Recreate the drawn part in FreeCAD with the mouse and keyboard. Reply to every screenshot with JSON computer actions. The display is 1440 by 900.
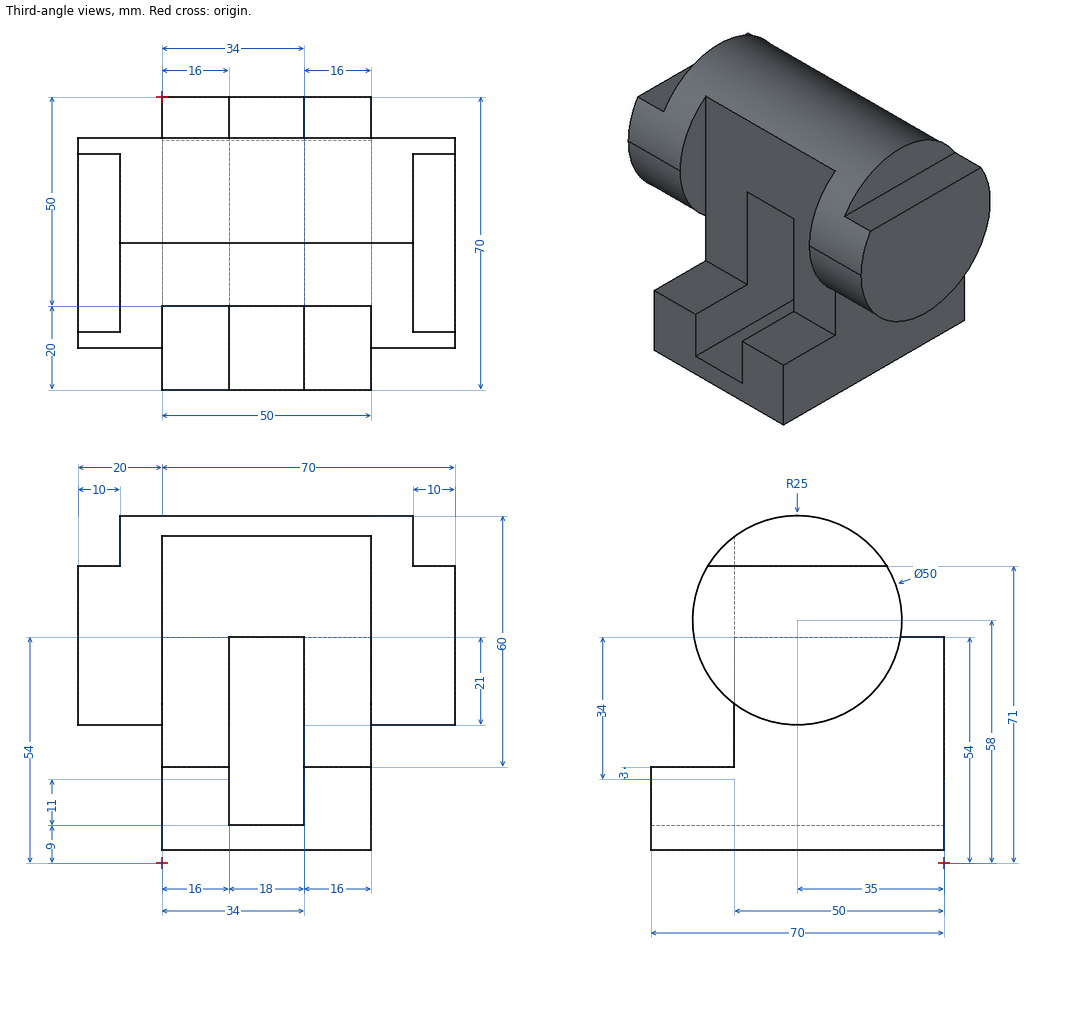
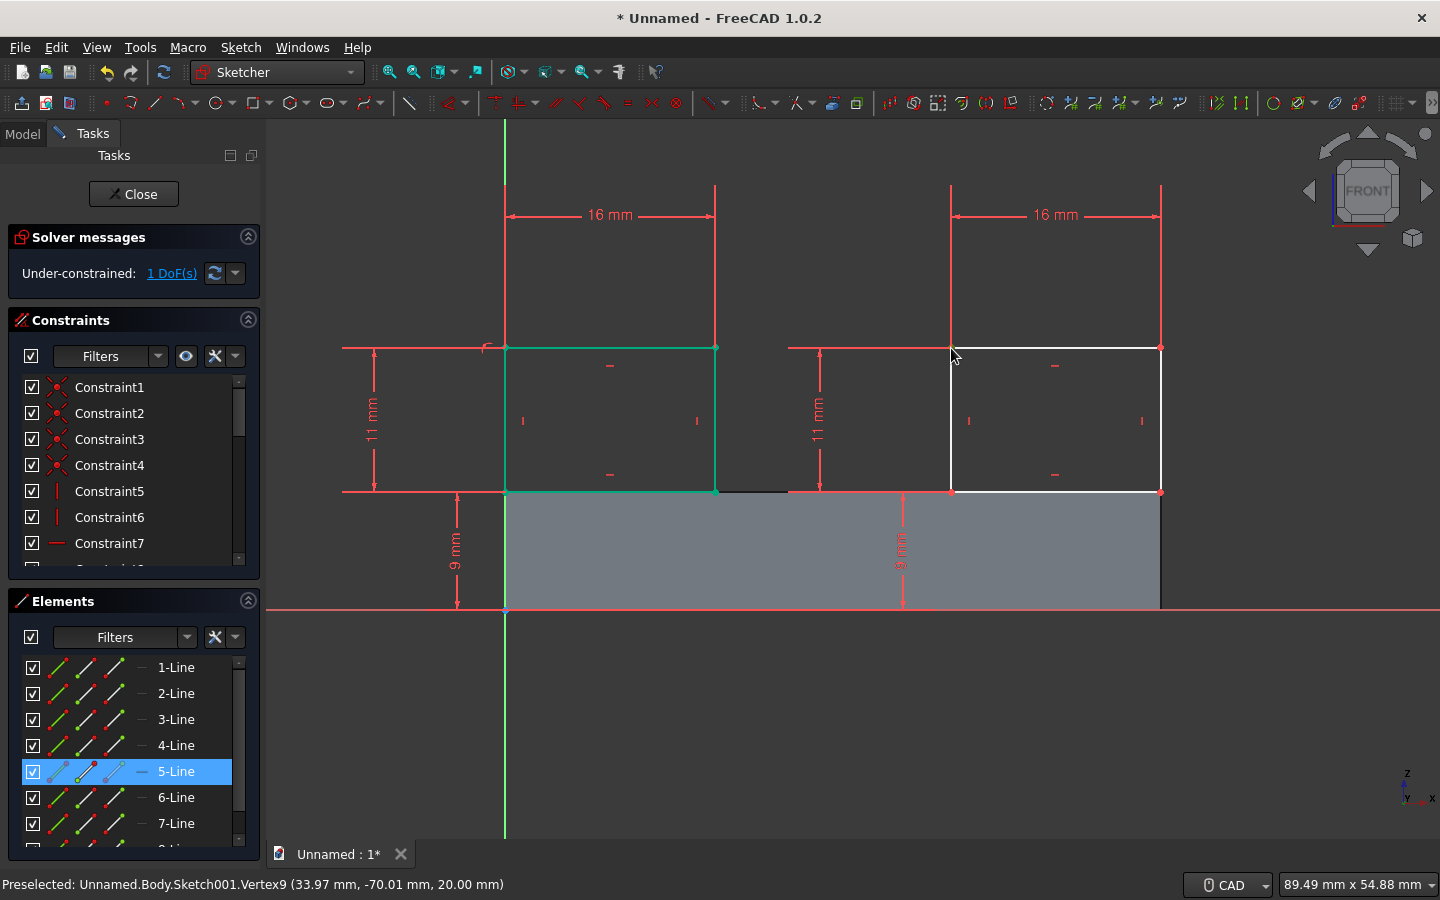
{"action": "key", "text": "l"}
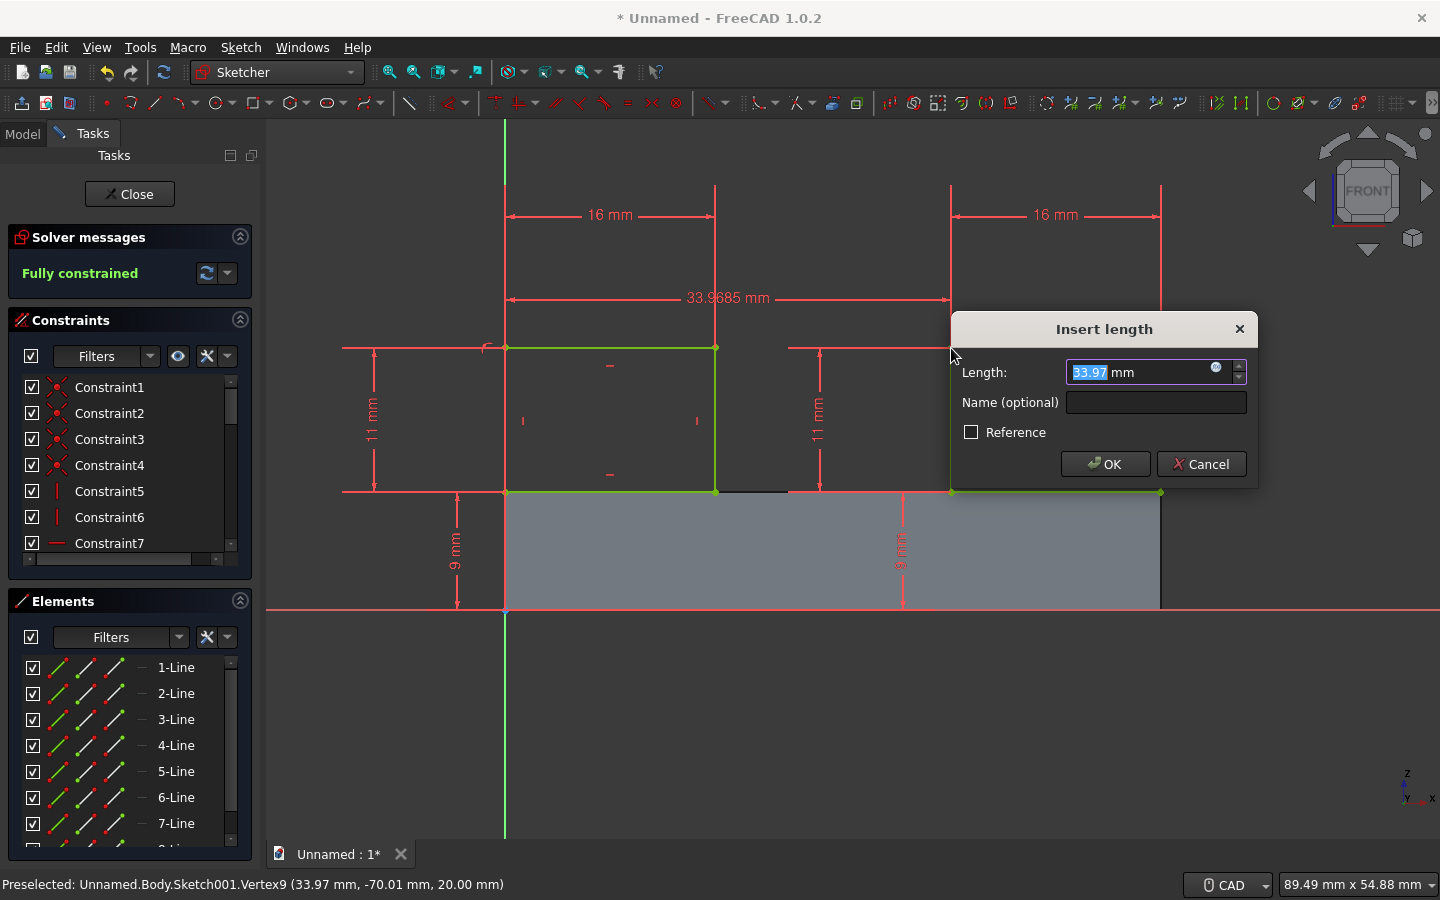
{"action": "type", "text": "34"}
{"action": "key", "text": "Return"}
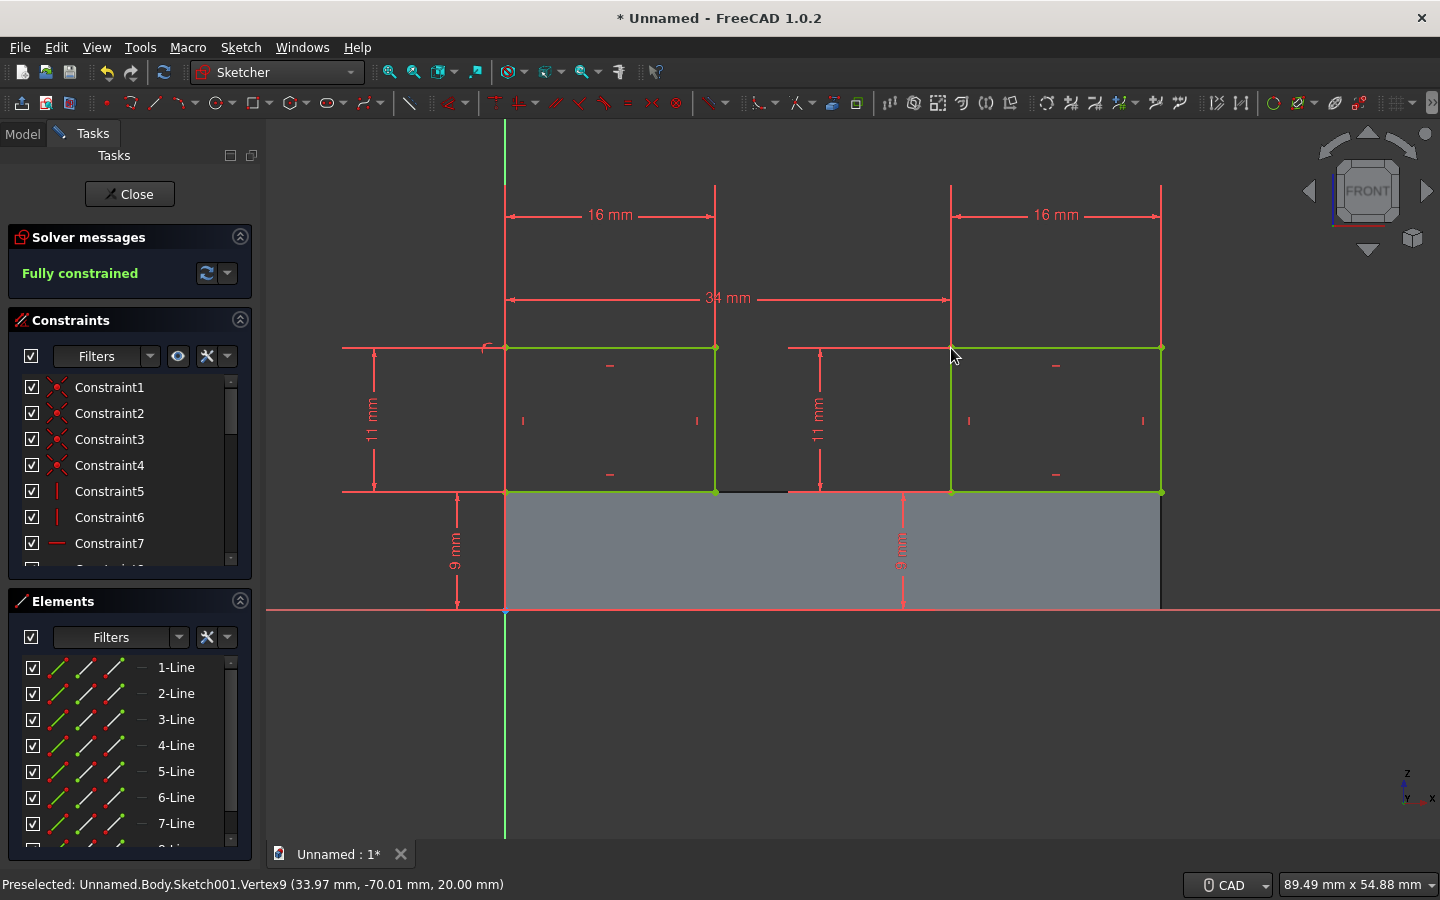
{"action": "left_click", "coordinate": [130, 194]}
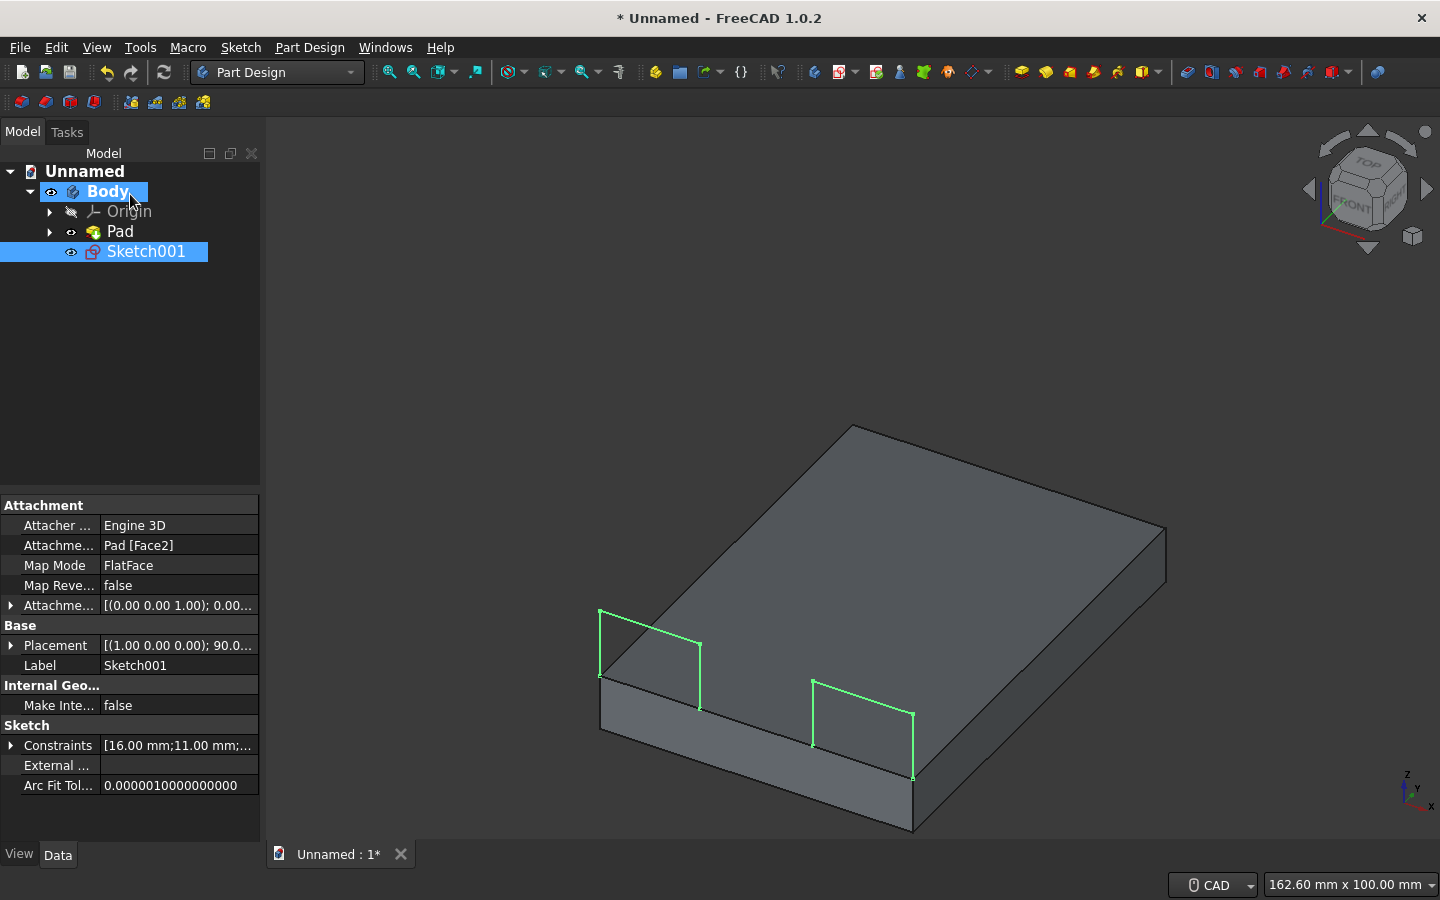
{"action": "left_click", "coordinate": [1022, 72]}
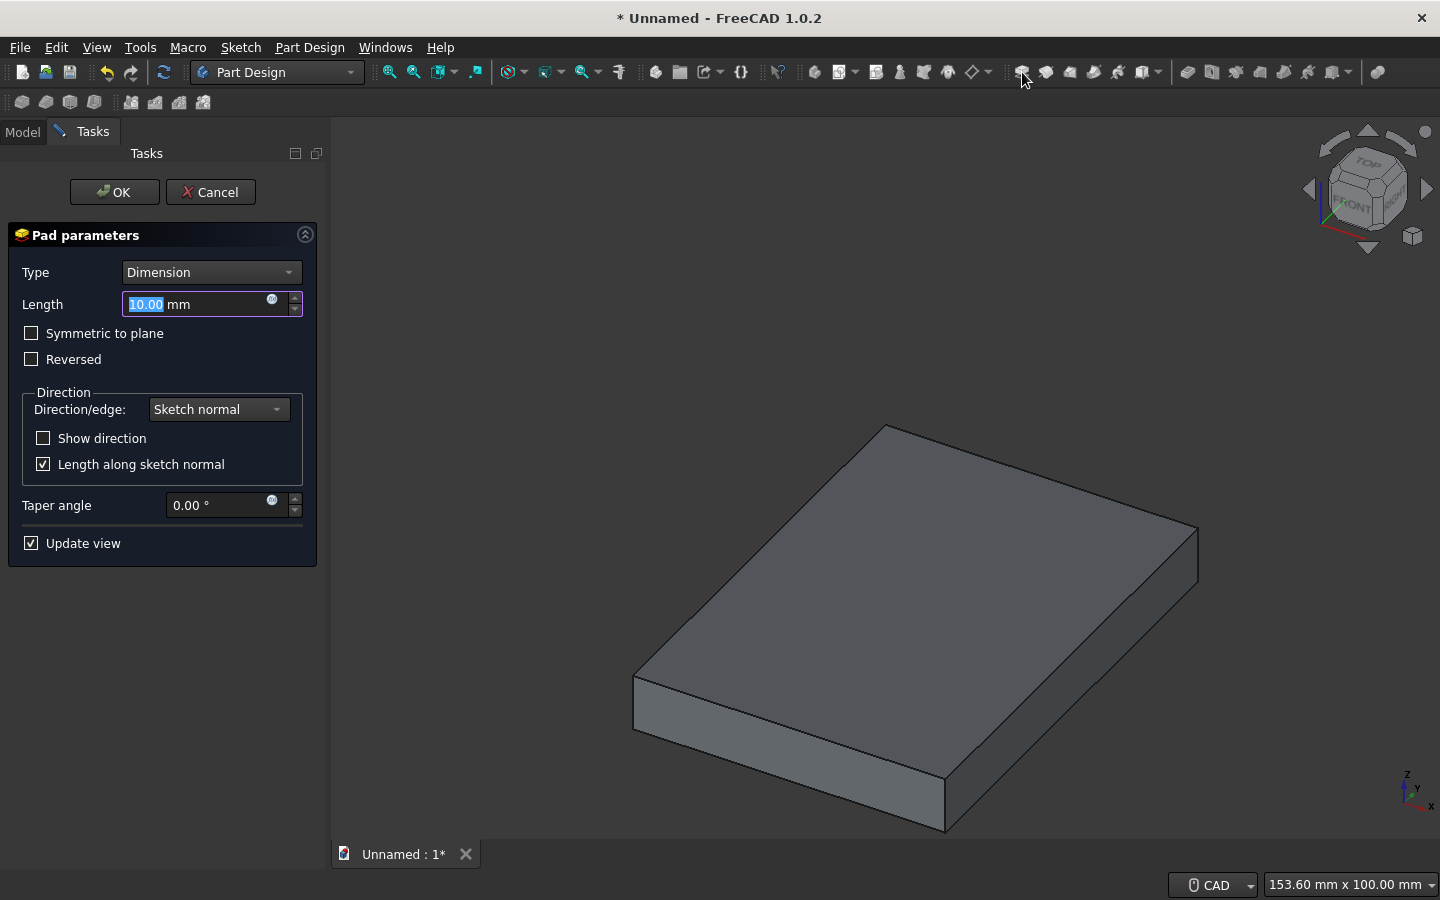
{"action": "type", "text": "70"}
{"action": "key", "text": "Tab"}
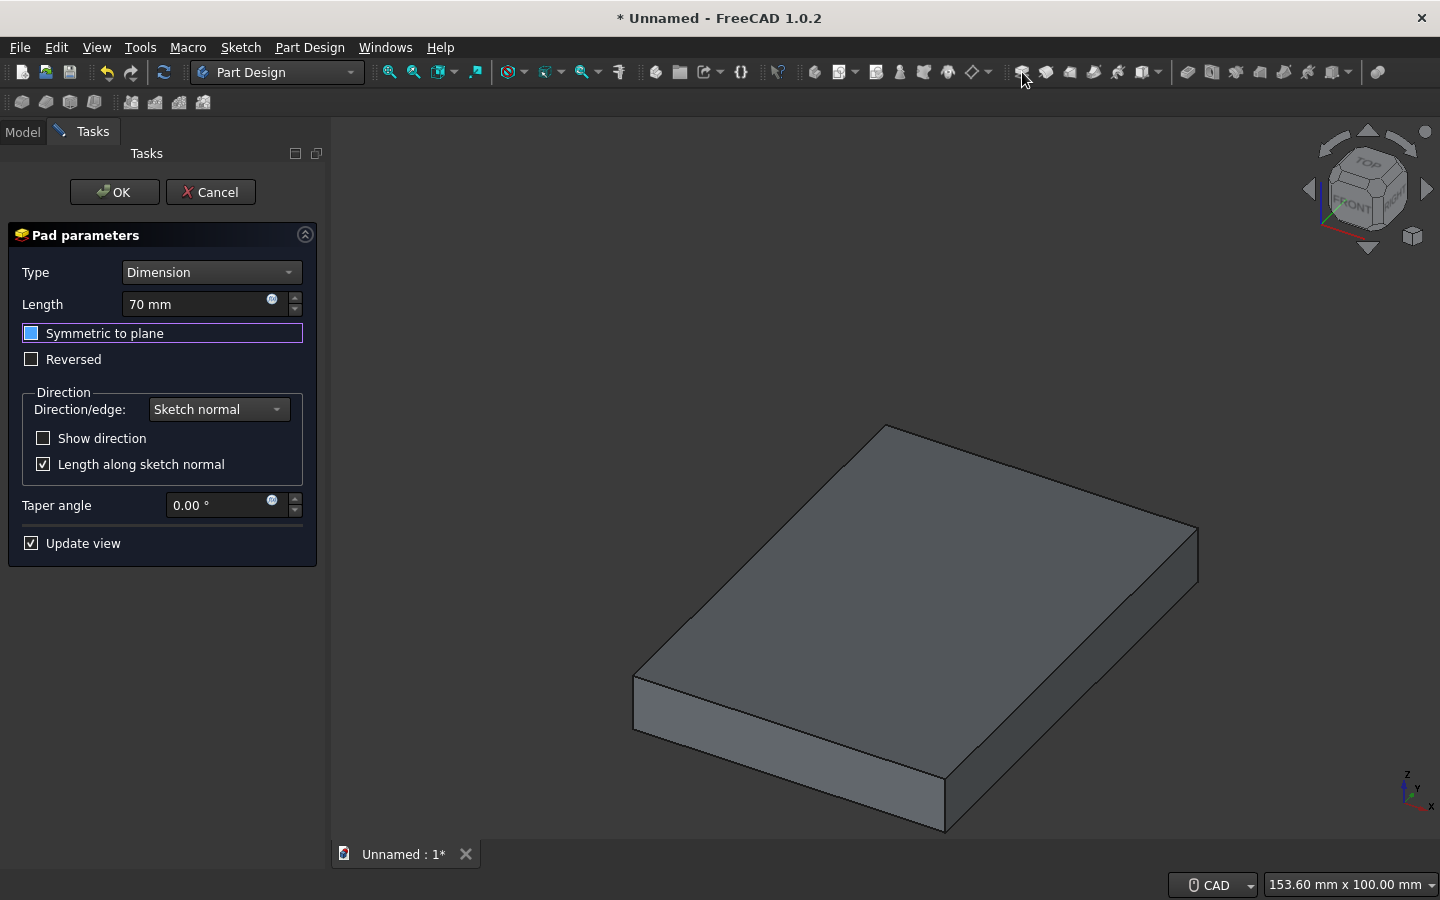
{"action": "left_click", "coordinate": [30, 359]}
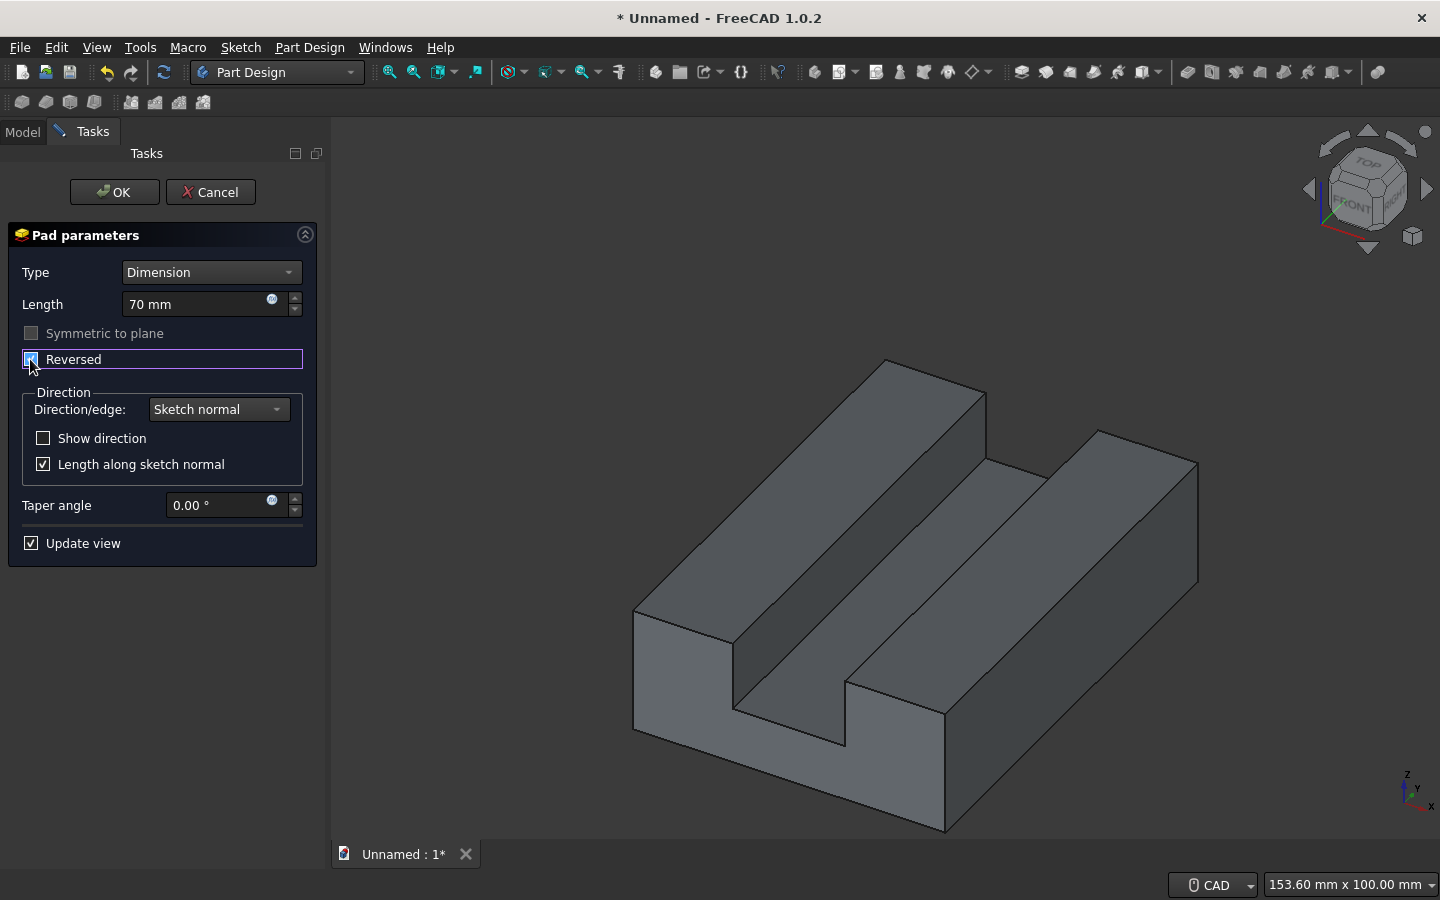
{"action": "left_click", "coordinate": [115, 192]}